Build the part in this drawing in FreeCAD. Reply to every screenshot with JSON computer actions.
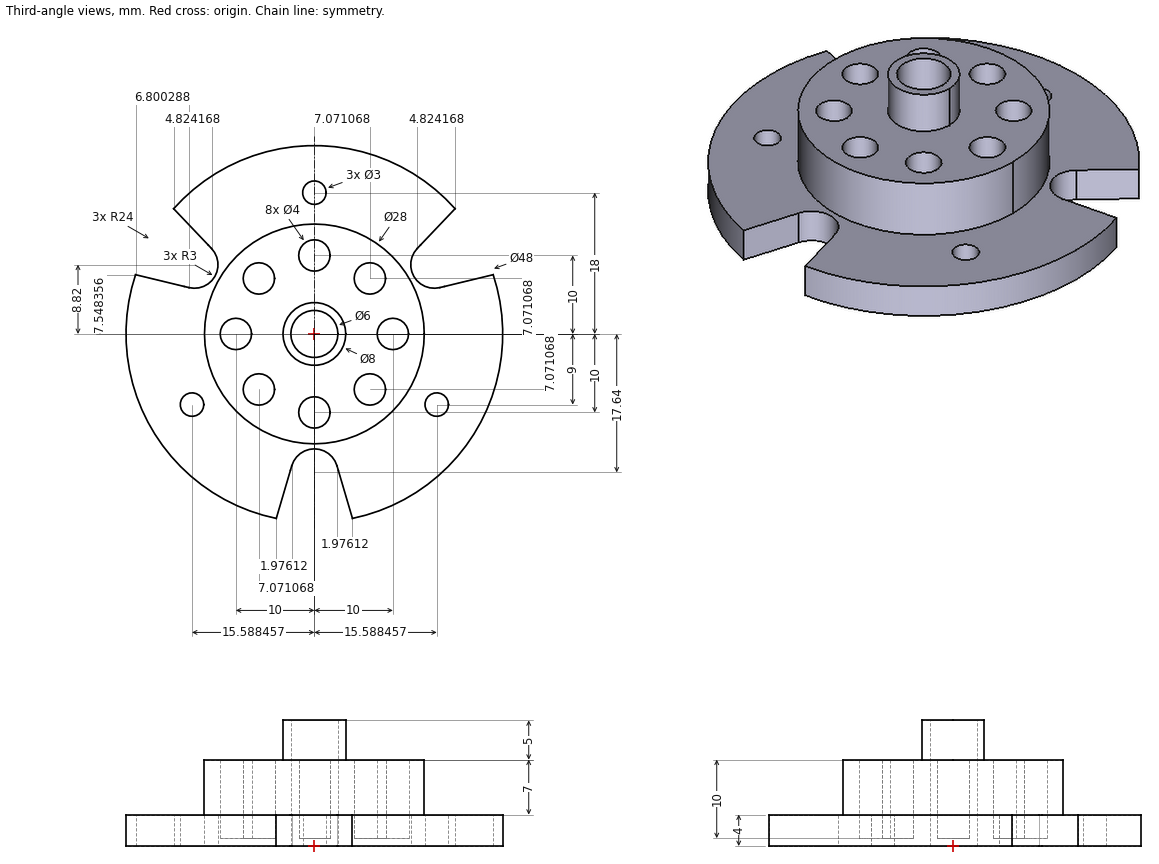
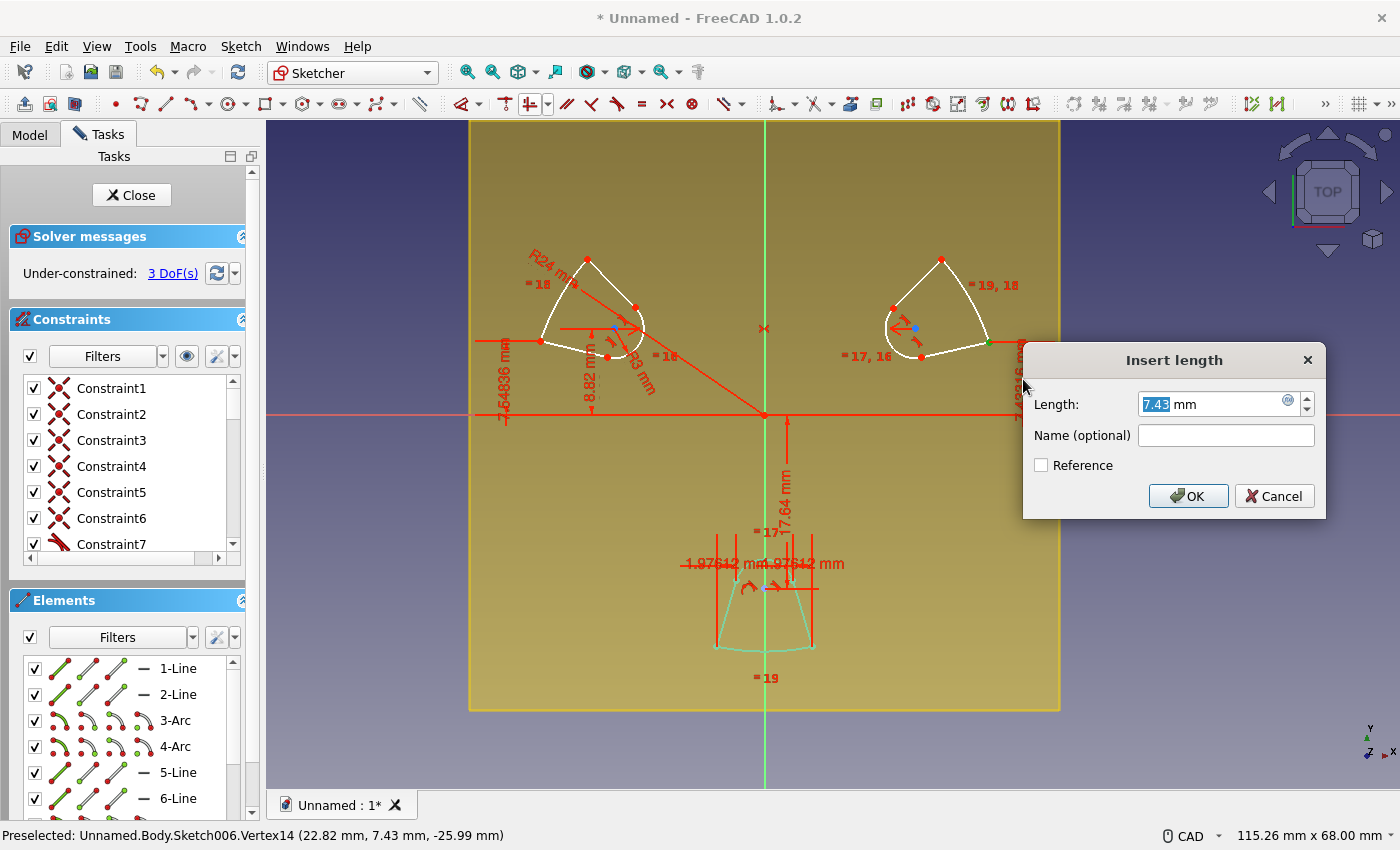
{"action": "type", "text": "7.548356"}
{"action": "key", "text": "Return"}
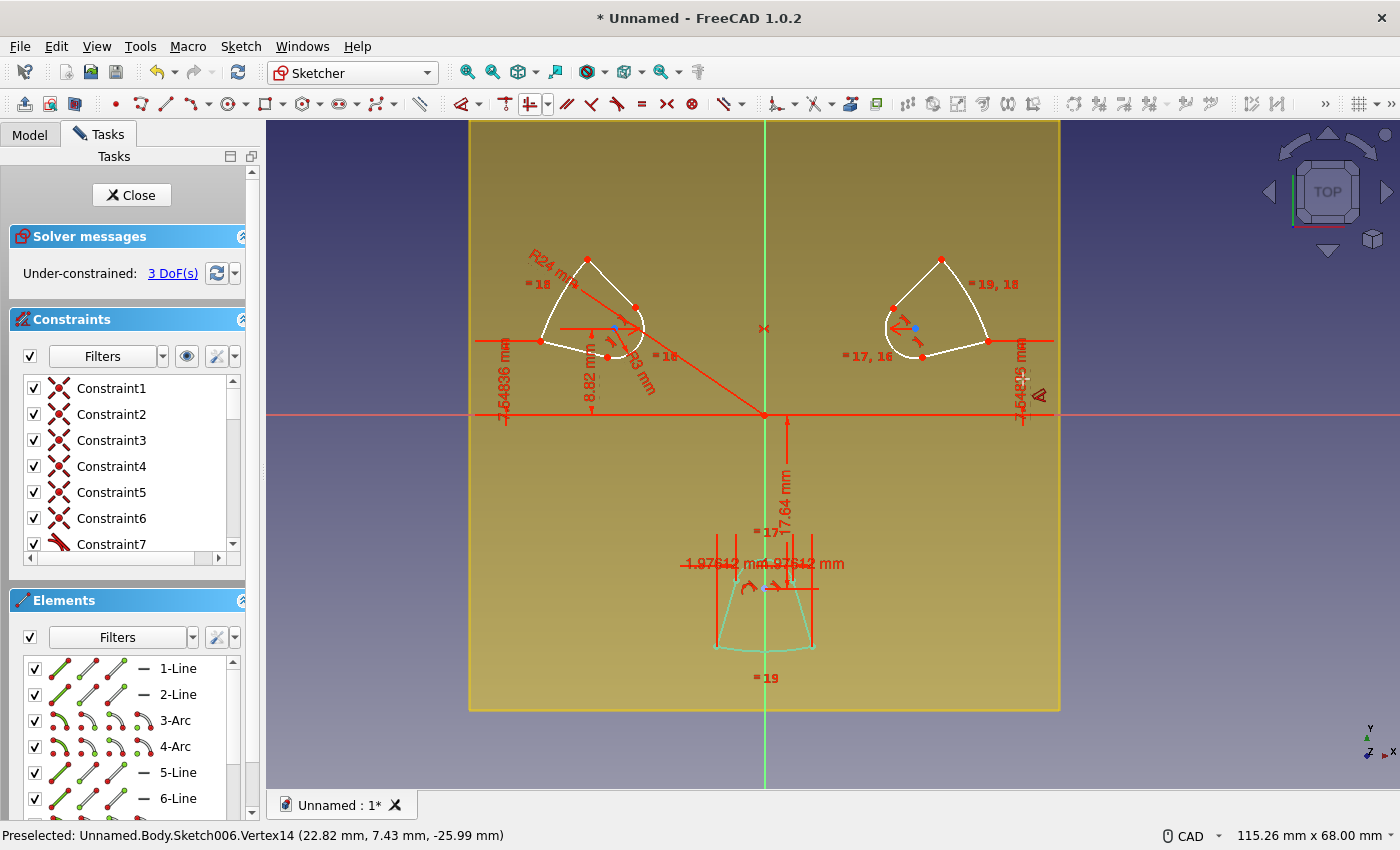
{"action": "left_click", "coordinate": [561, 346]}
{"action": "left_click", "coordinate": [574, 307]}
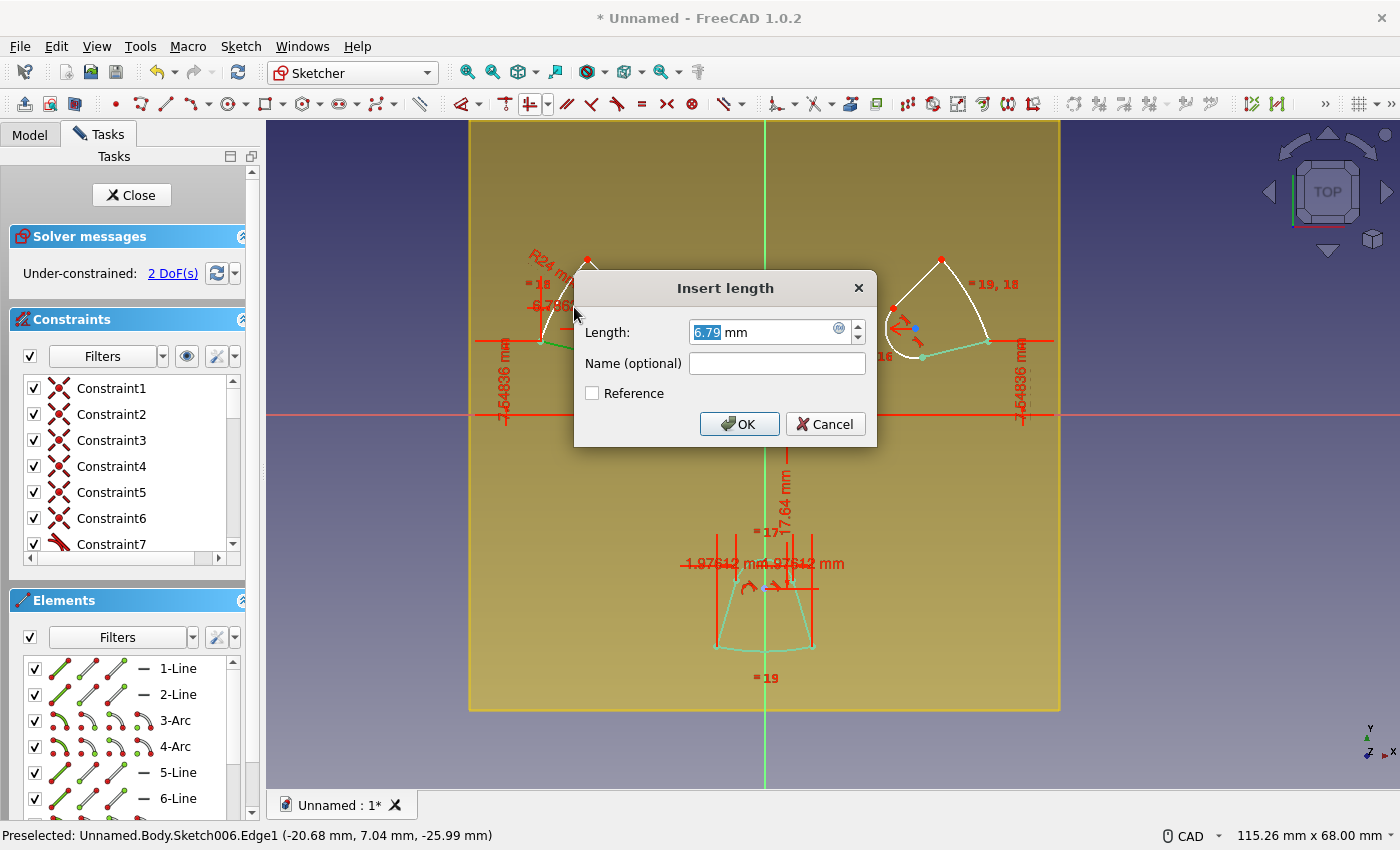
{"action": "type", "text": "6.800288"}
{"action": "key", "text": "Return"}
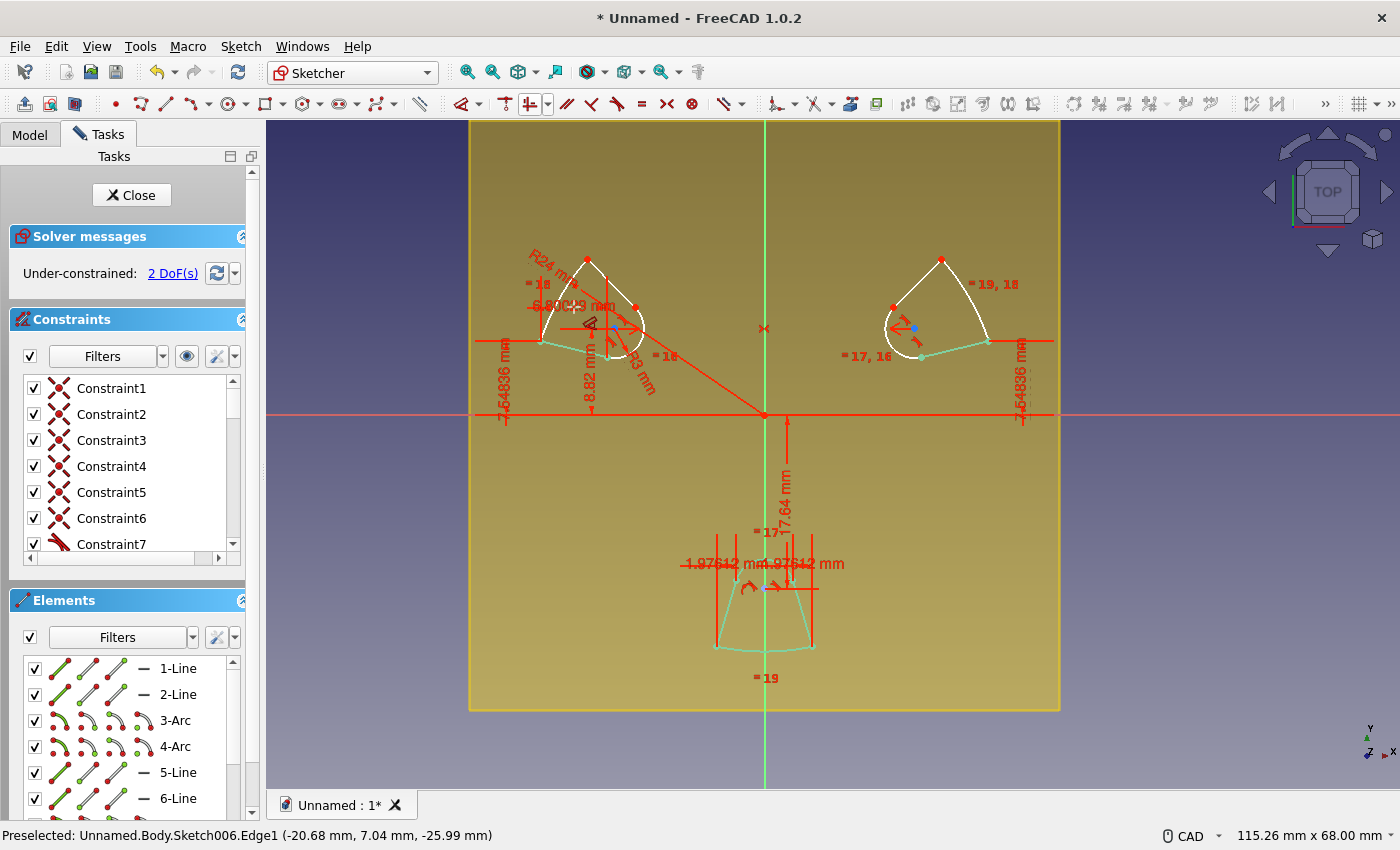
{"action": "left_click", "coordinate": [621, 293]}
{"action": "left_click", "coordinate": [611, 225]}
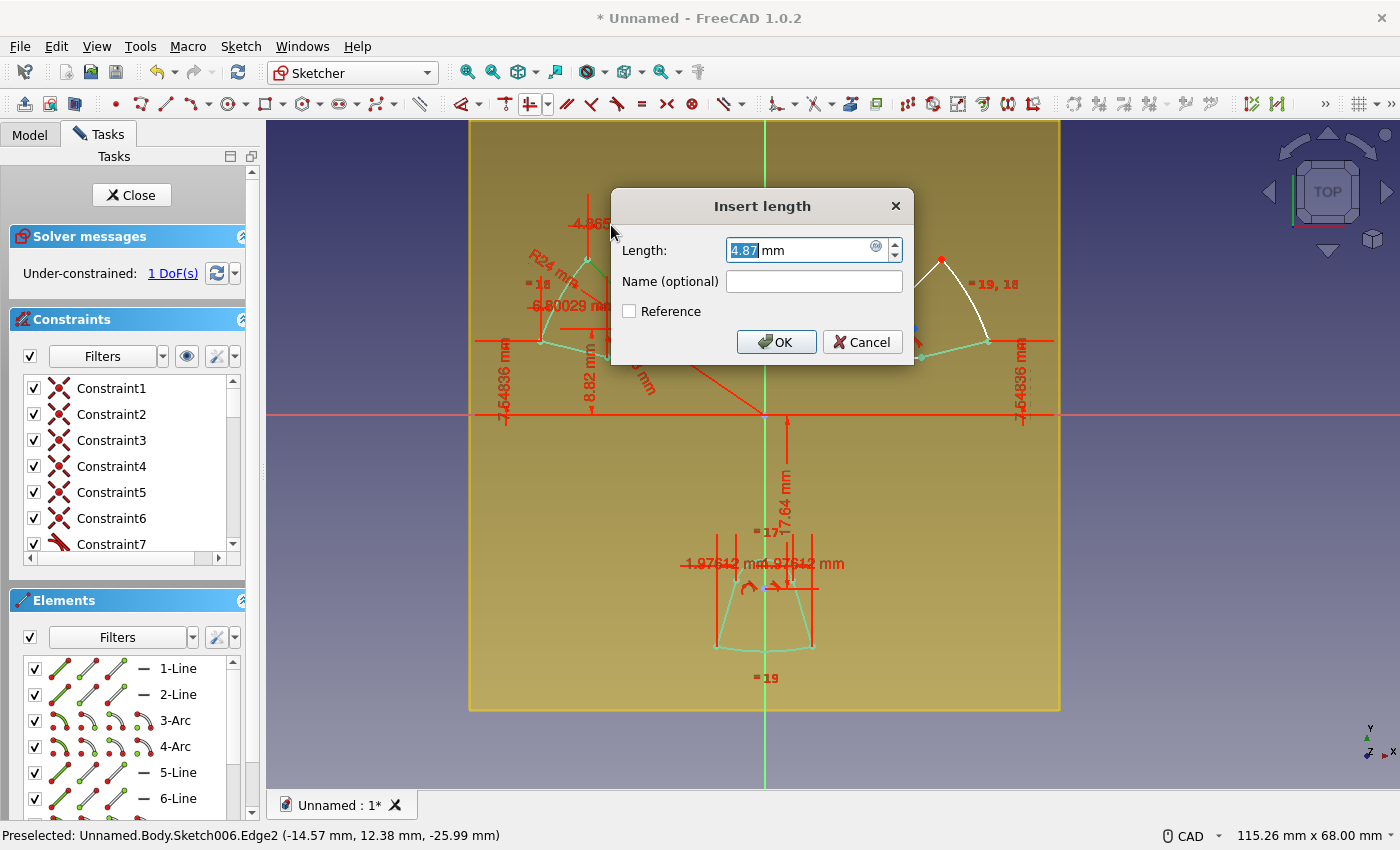
{"action": "type", "text": "4.824168"}
{"action": "key", "text": "Return"}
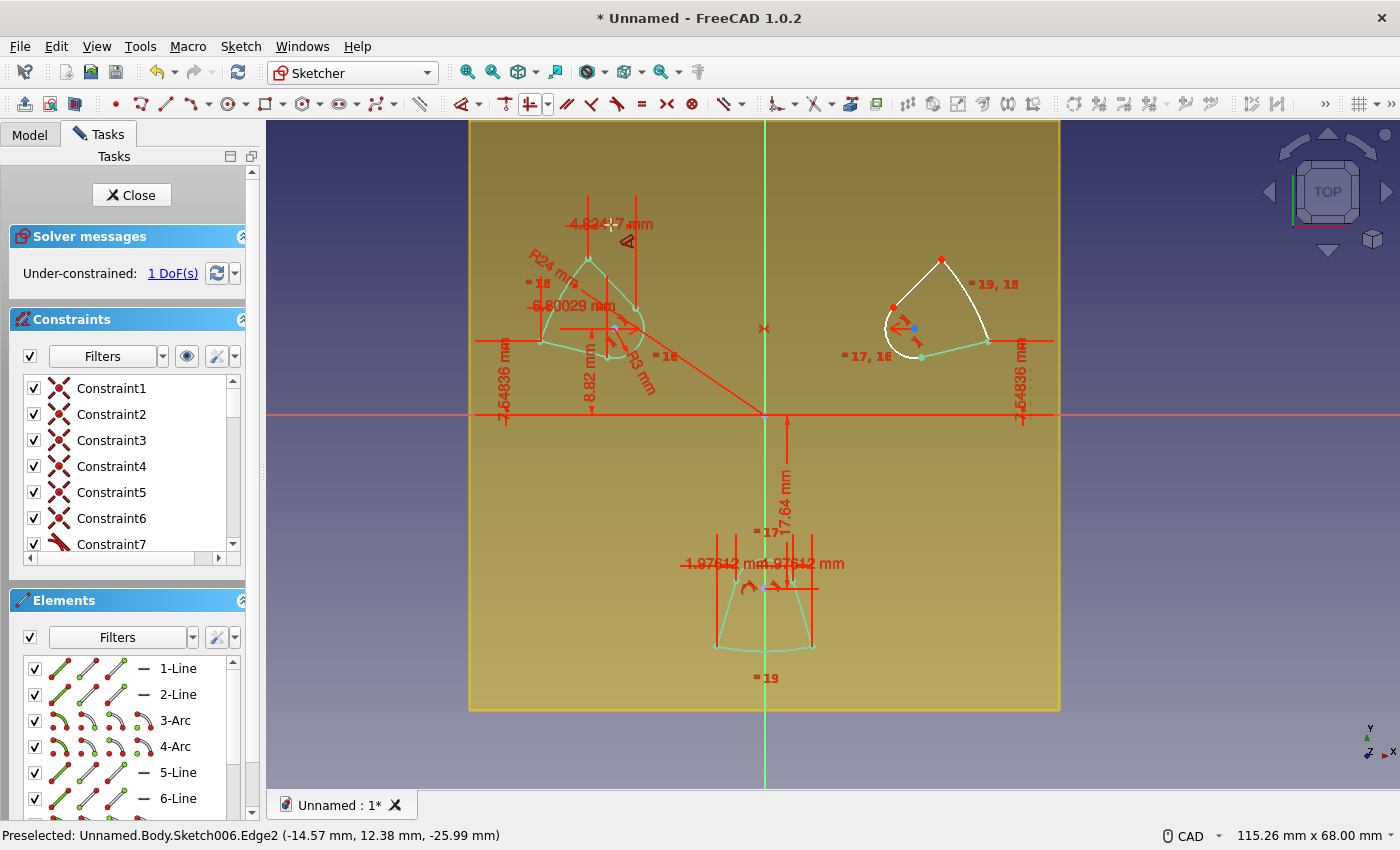
{"action": "left_click", "coordinate": [927, 274]}
{"action": "left_click", "coordinate": [918, 225]}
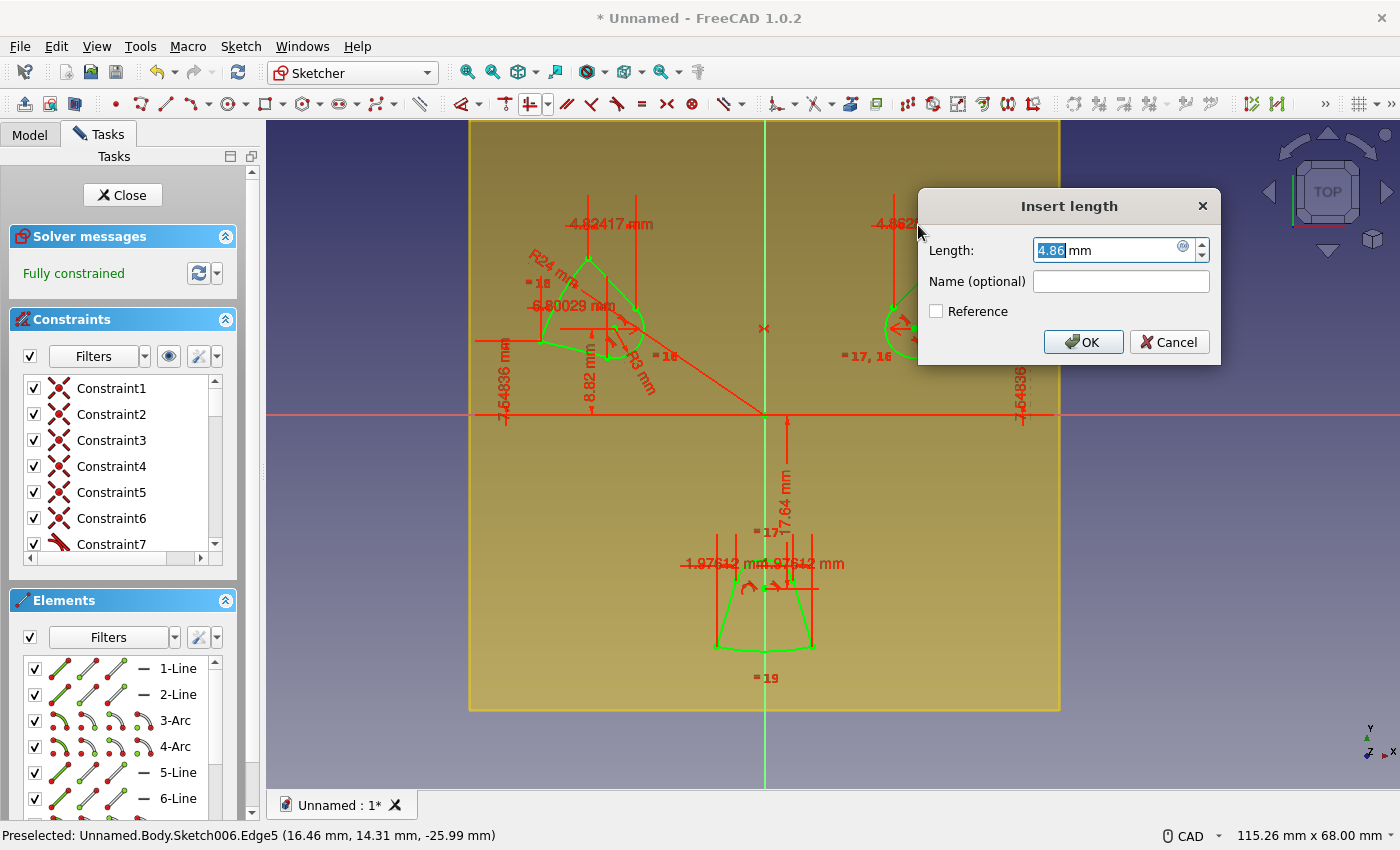
{"action": "type", "text": "4.824168"}
{"action": "key", "text": "Return"}
{"action": "key", "text": "Escape"}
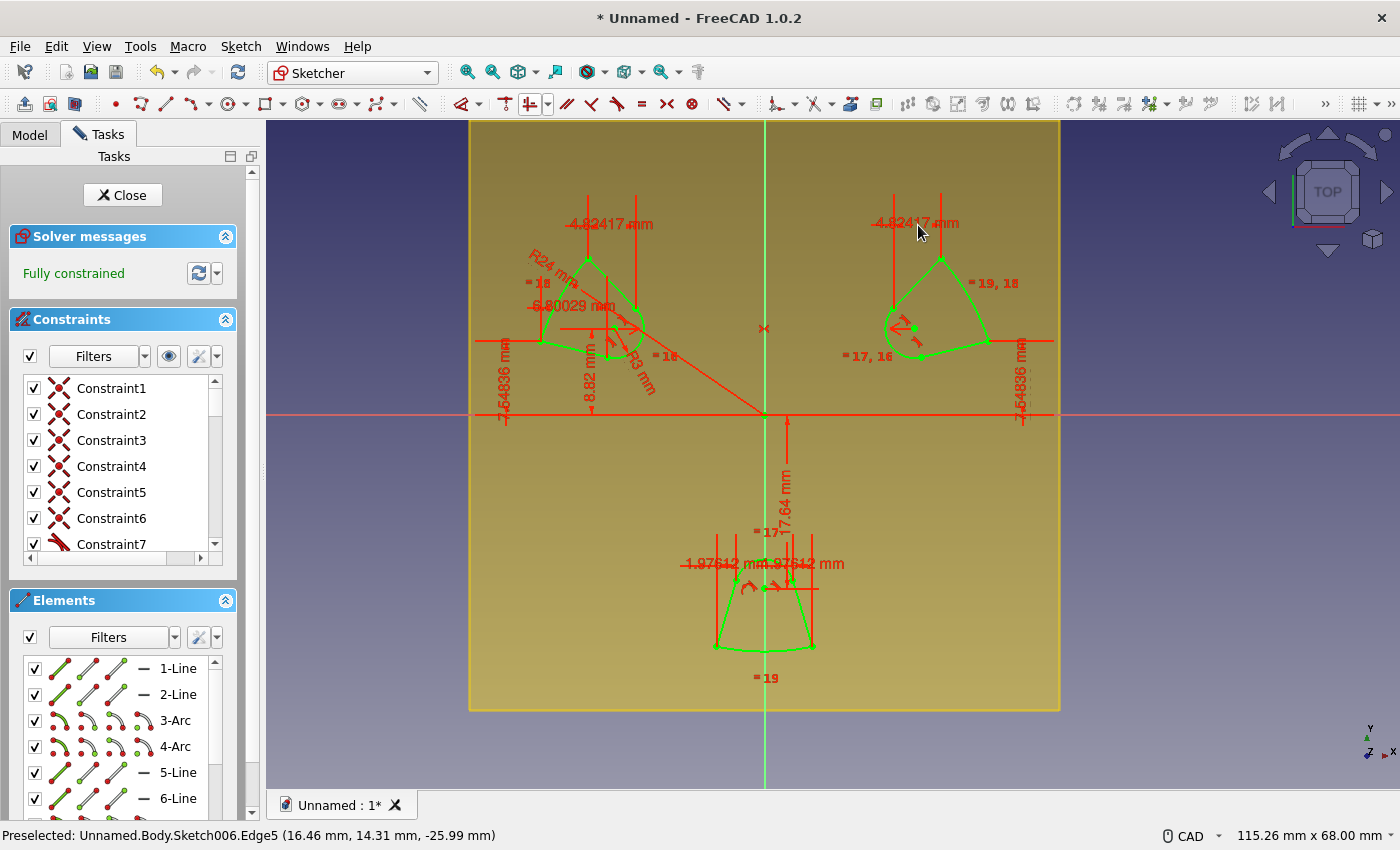
{"action": "left_click", "coordinate": [123, 195]}